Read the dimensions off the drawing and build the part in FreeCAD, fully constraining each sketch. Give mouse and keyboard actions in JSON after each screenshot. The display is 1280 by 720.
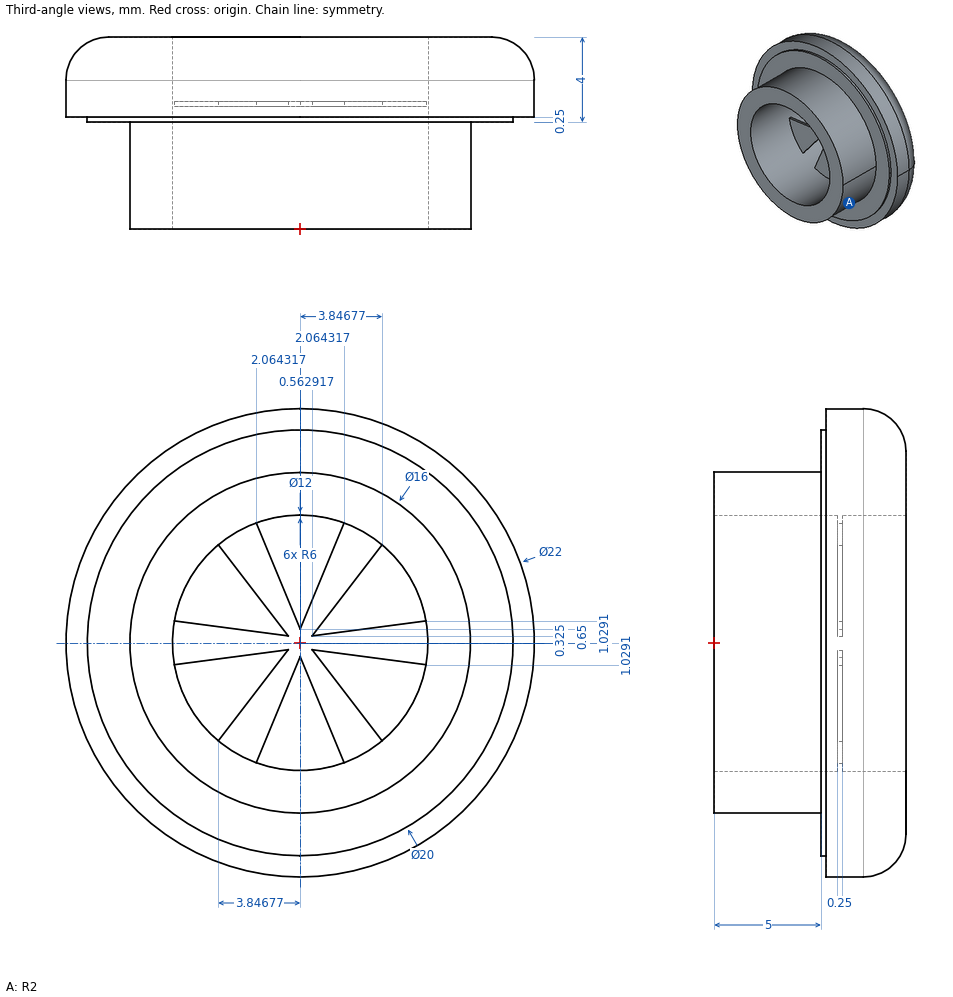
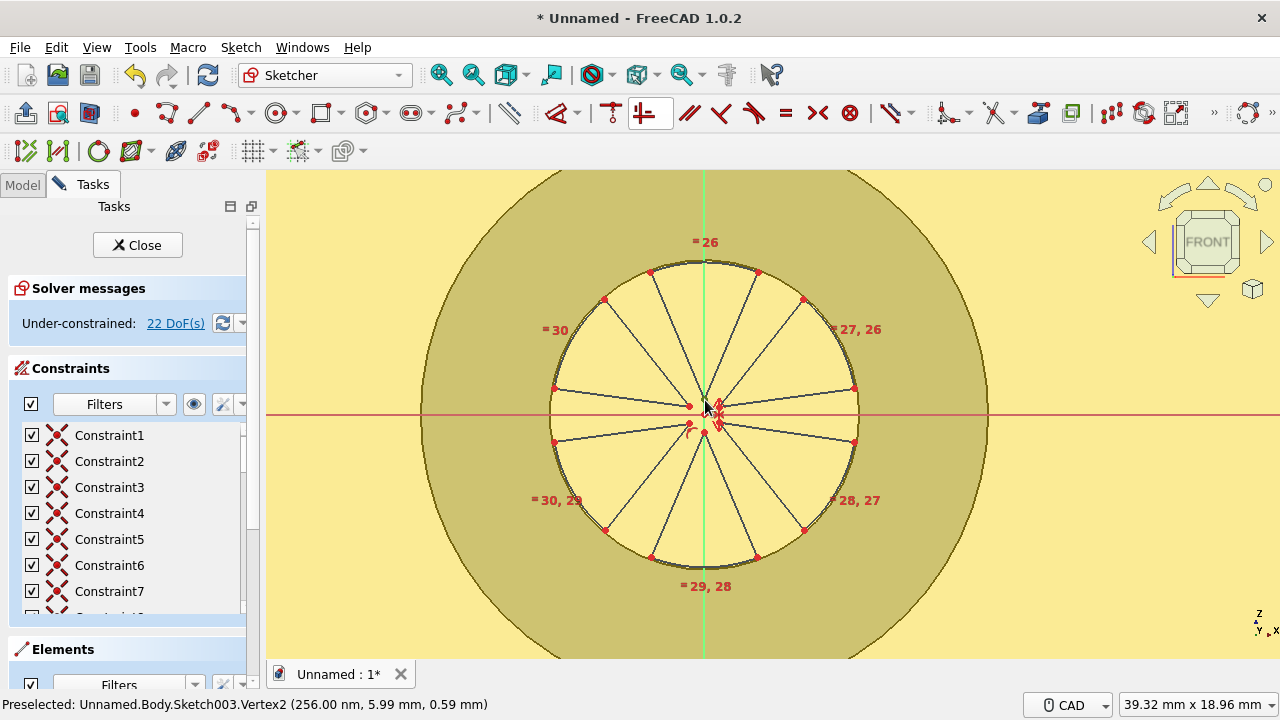
{"action": "left_click", "coordinate": [704, 432]}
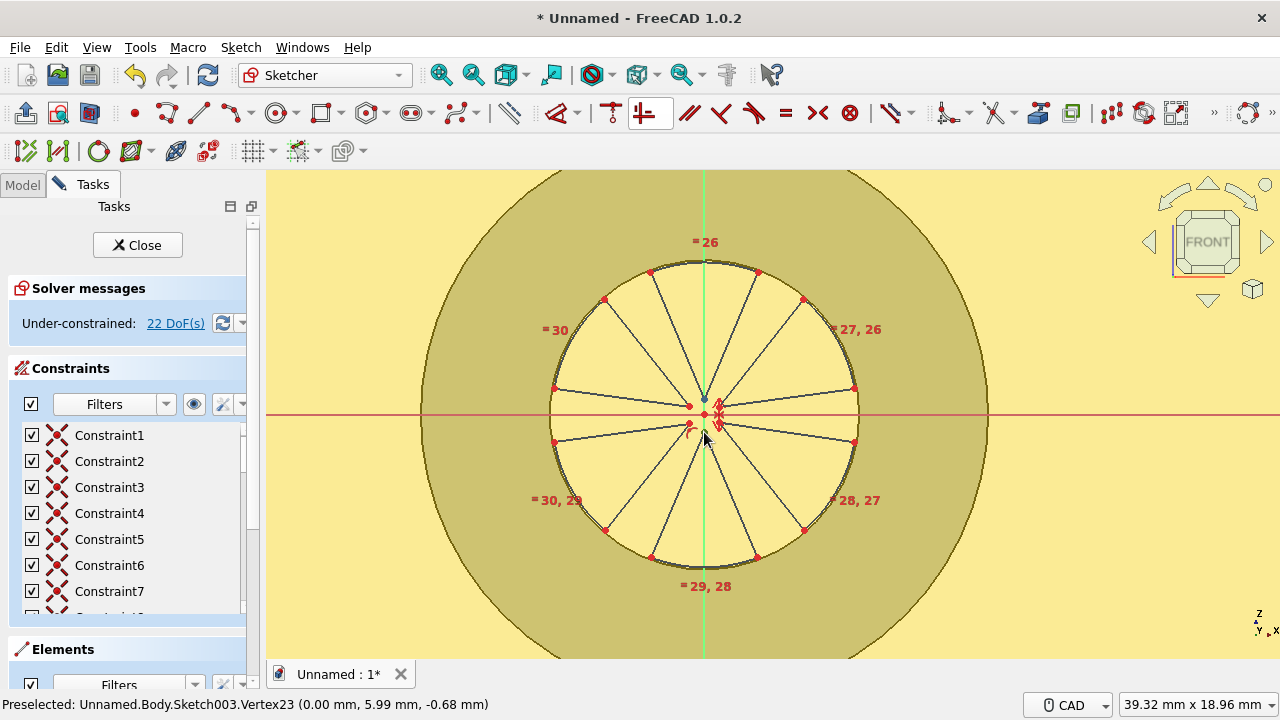
{"action": "left_click", "coordinate": [353, 415]}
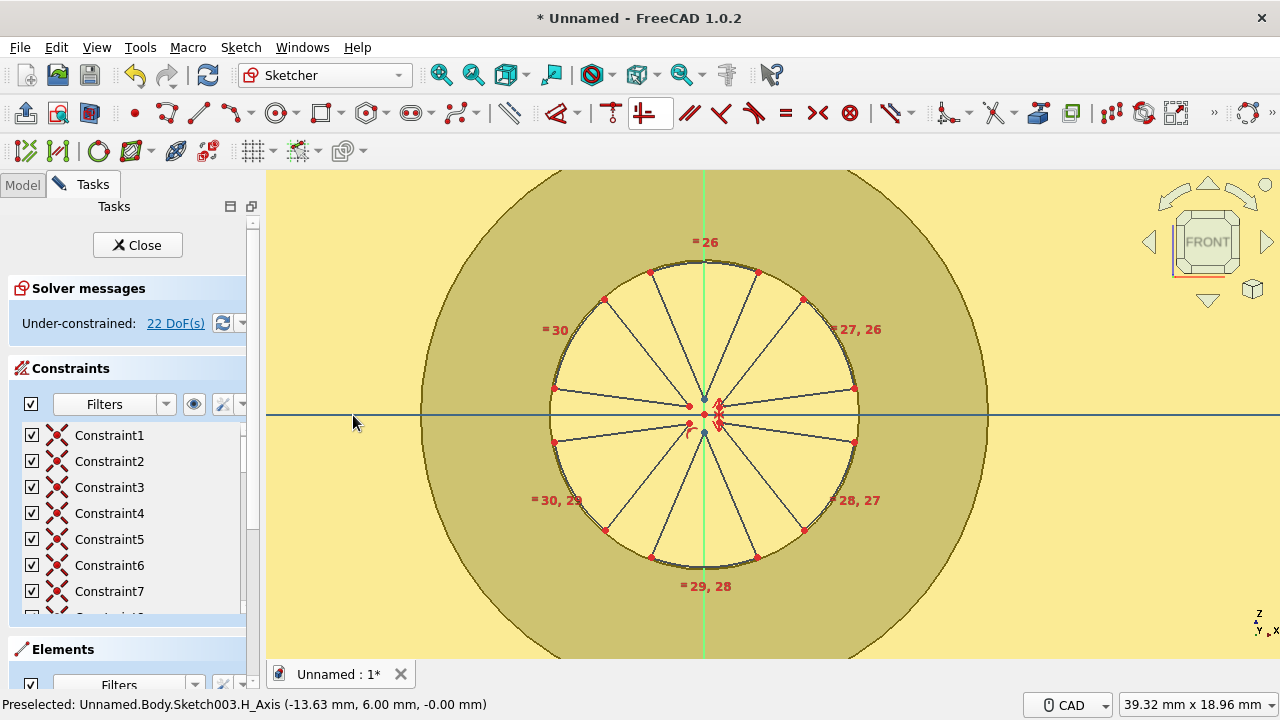
{"action": "key", "text": "s"}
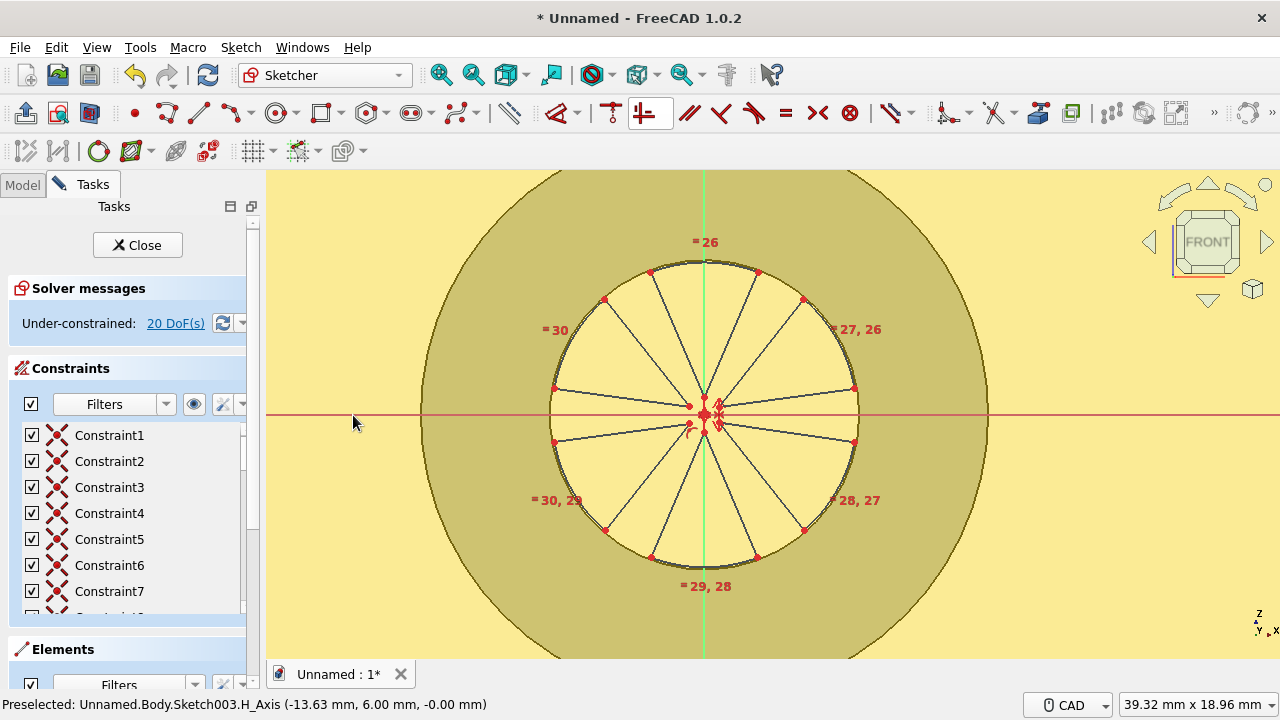
{"action": "left_click", "coordinate": [719, 423]}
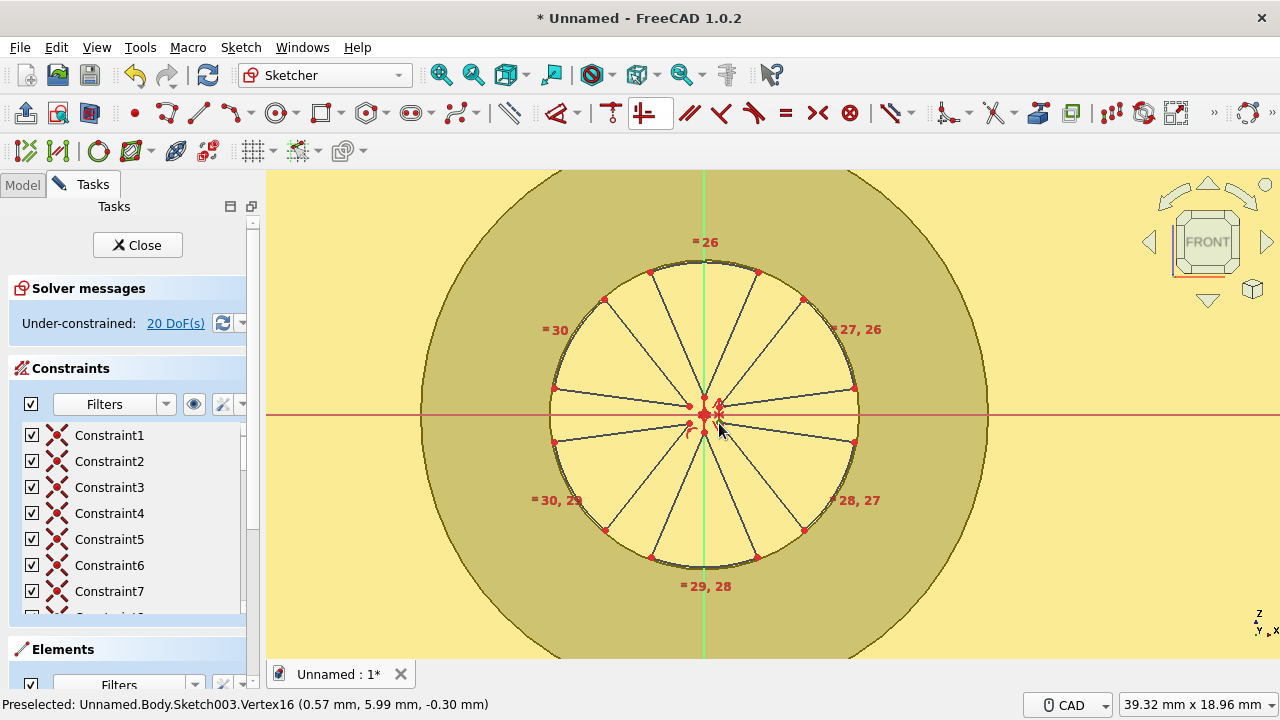
{"action": "left_click", "coordinate": [690, 424]}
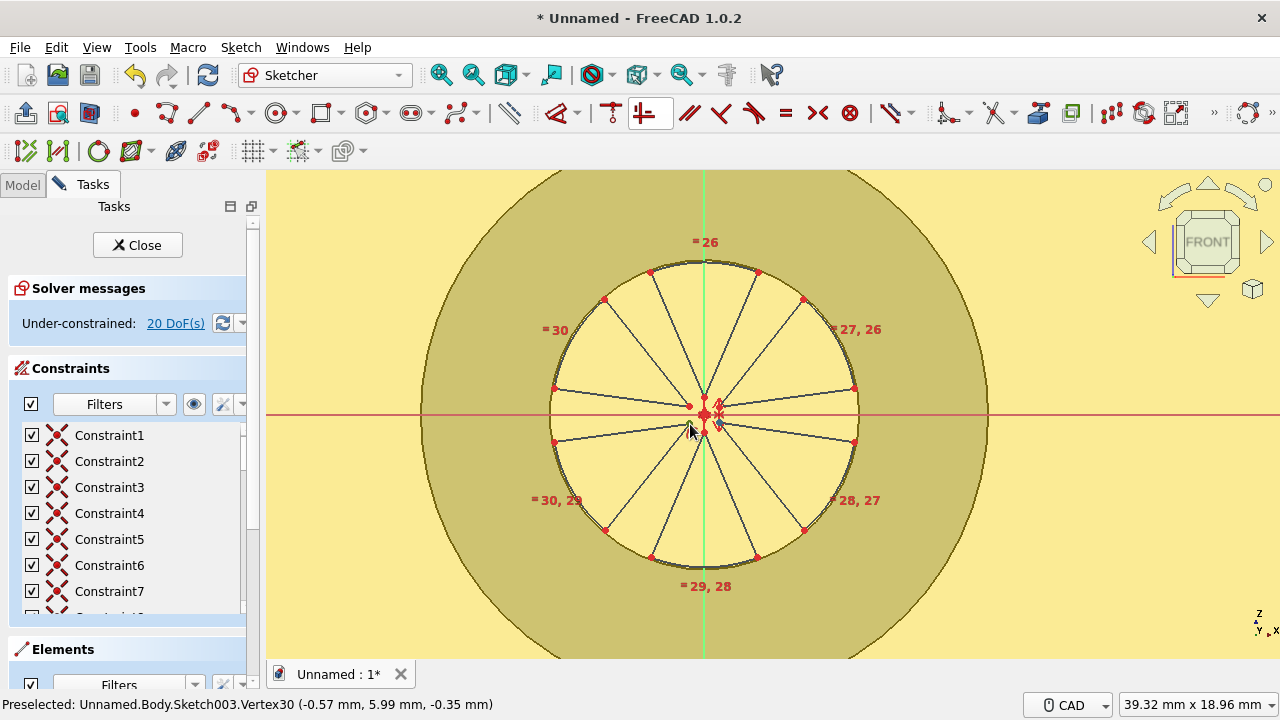
{"action": "left_click", "coordinate": [704, 600]}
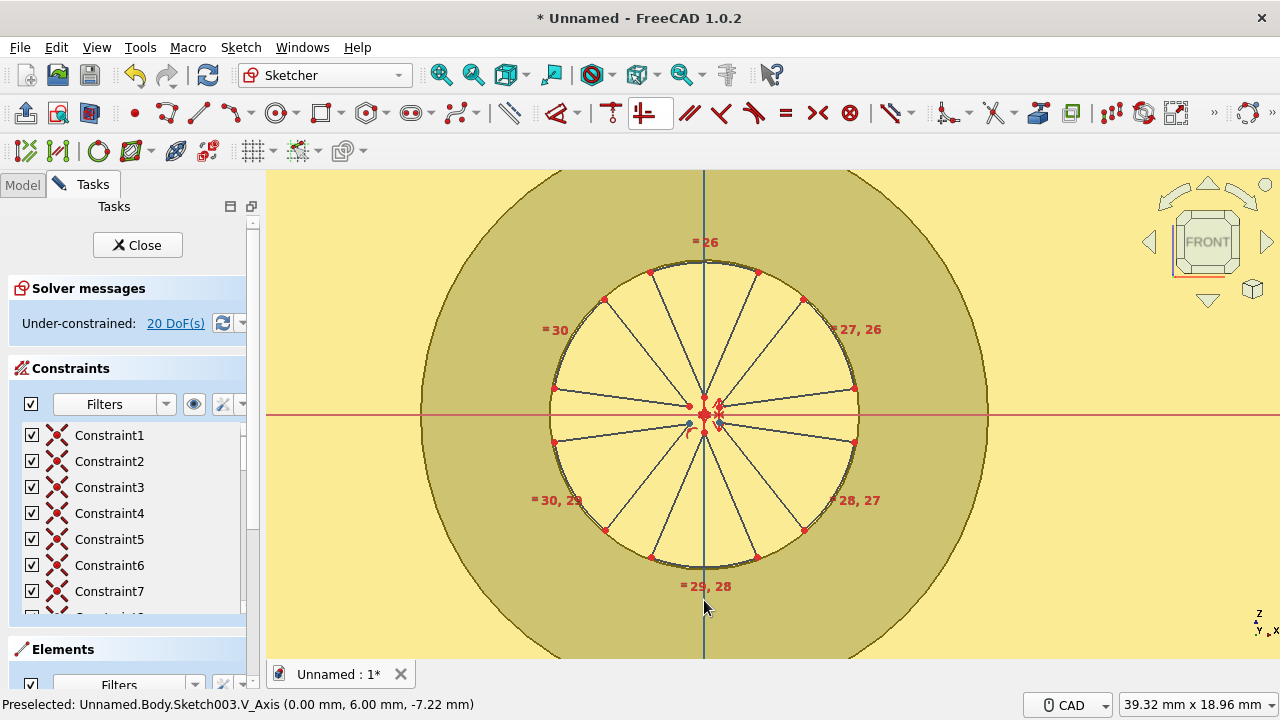
{"action": "key", "text": "s"}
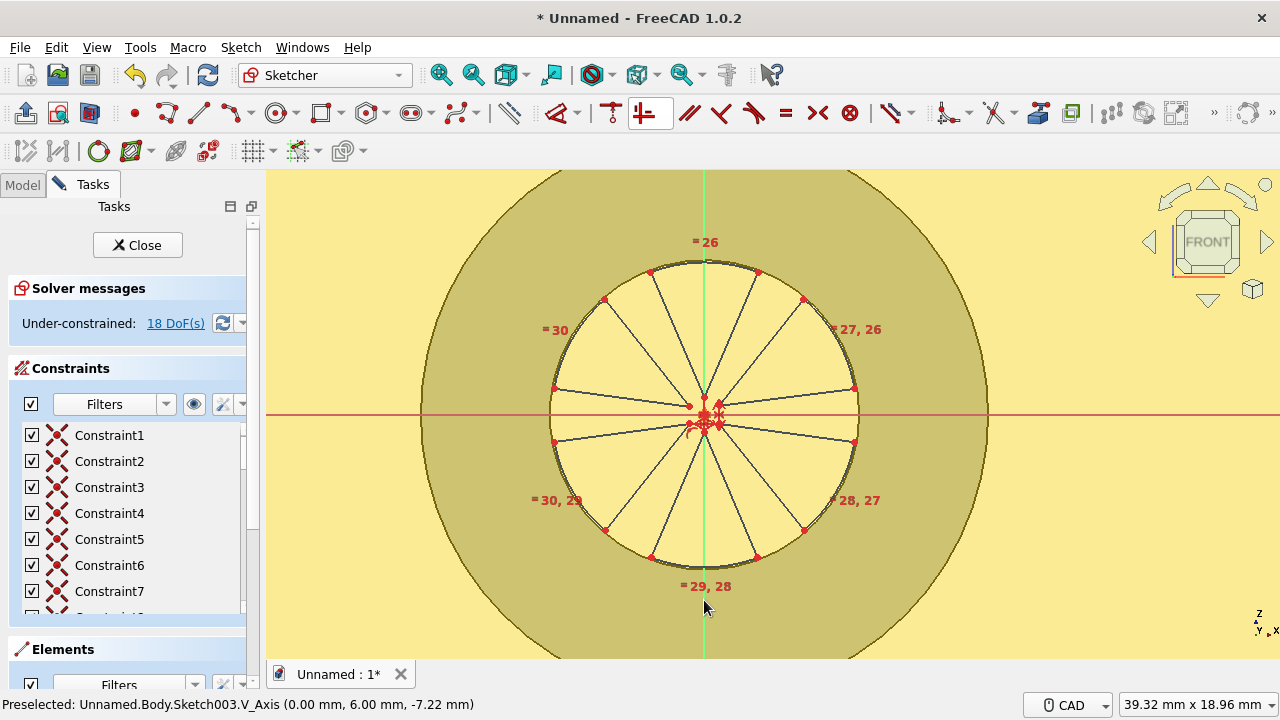
{"action": "left_click", "coordinate": [719, 406]}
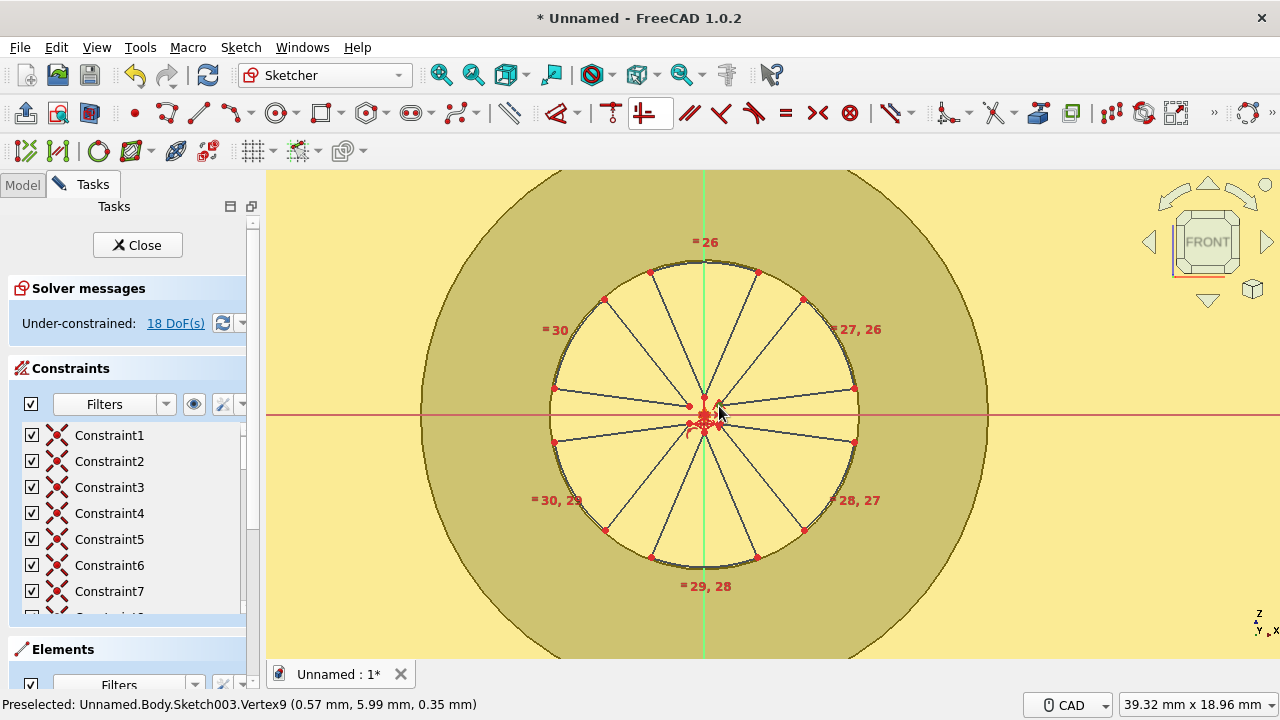
{"action": "left_click", "coordinate": [690, 407]}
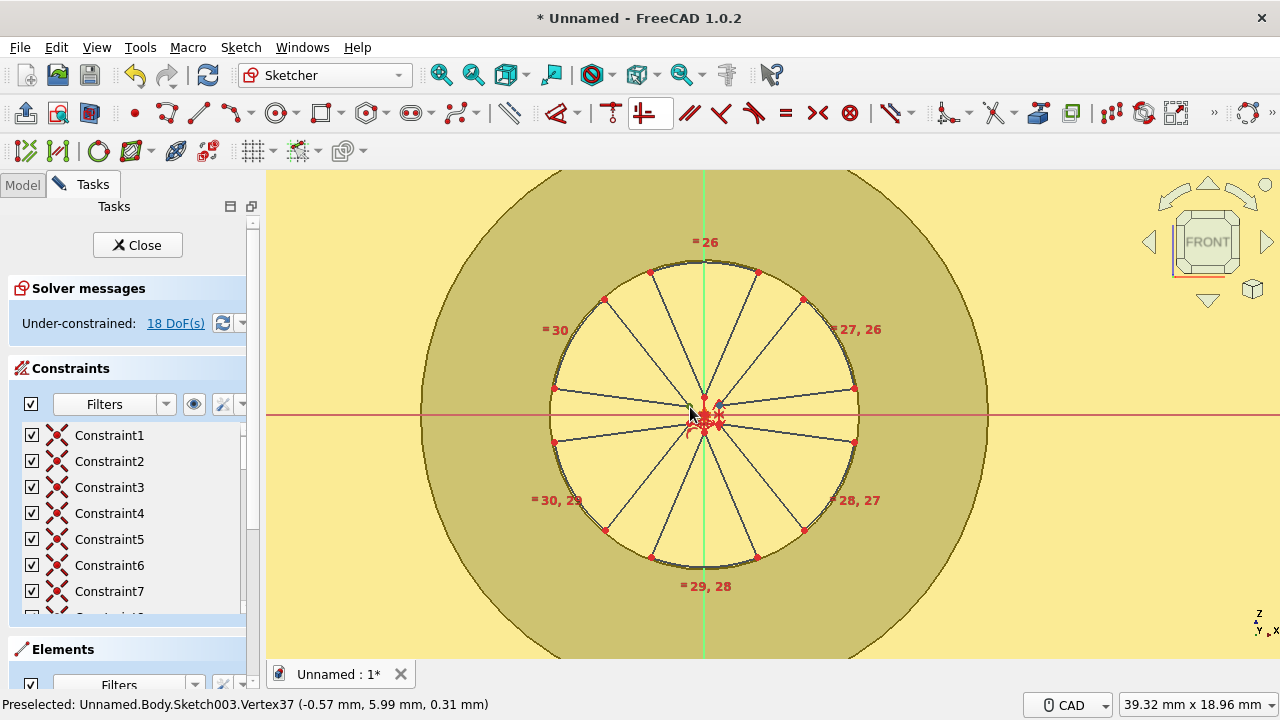
{"action": "left_click", "coordinate": [704, 600]}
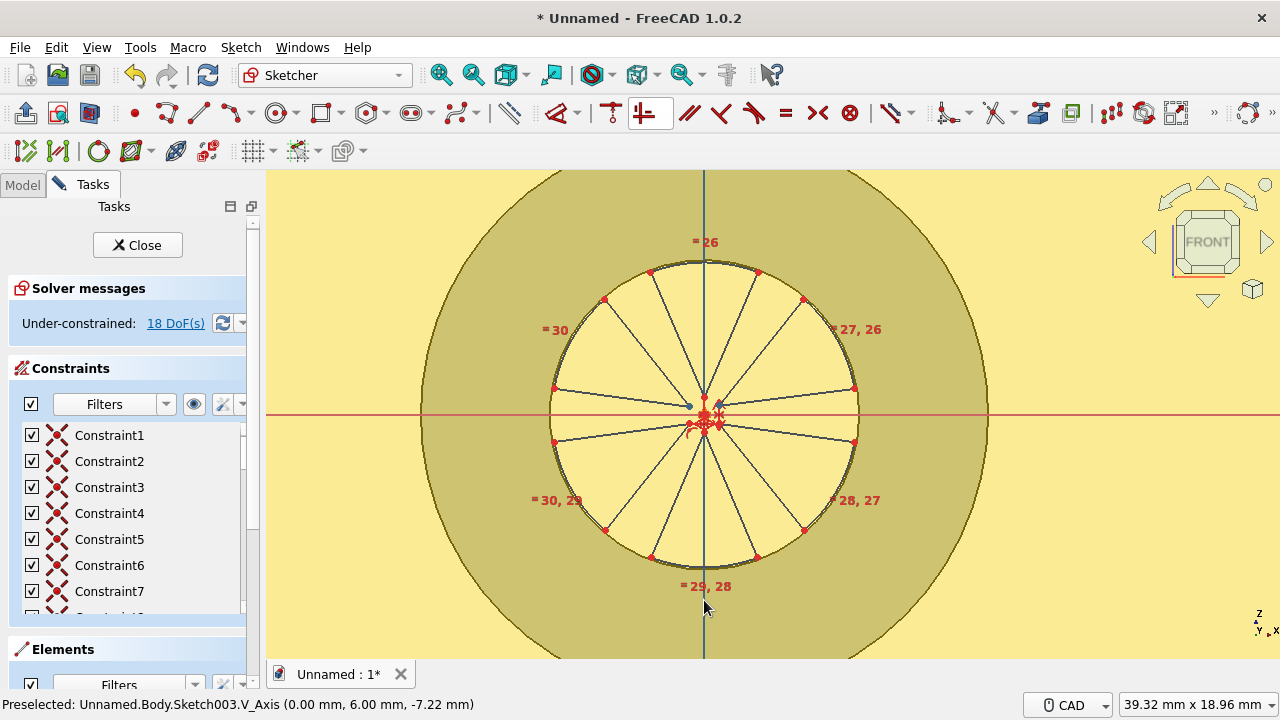
{"action": "key", "text": "s"}